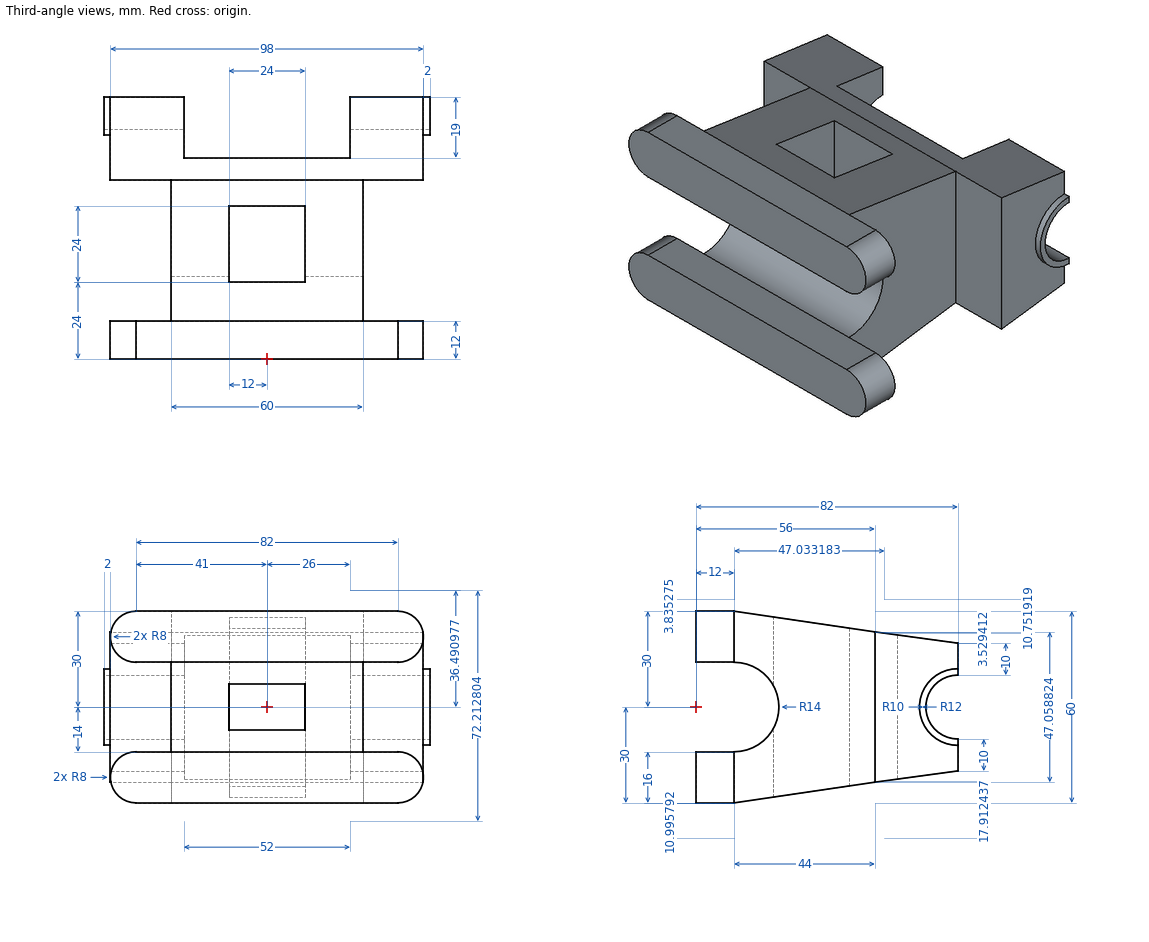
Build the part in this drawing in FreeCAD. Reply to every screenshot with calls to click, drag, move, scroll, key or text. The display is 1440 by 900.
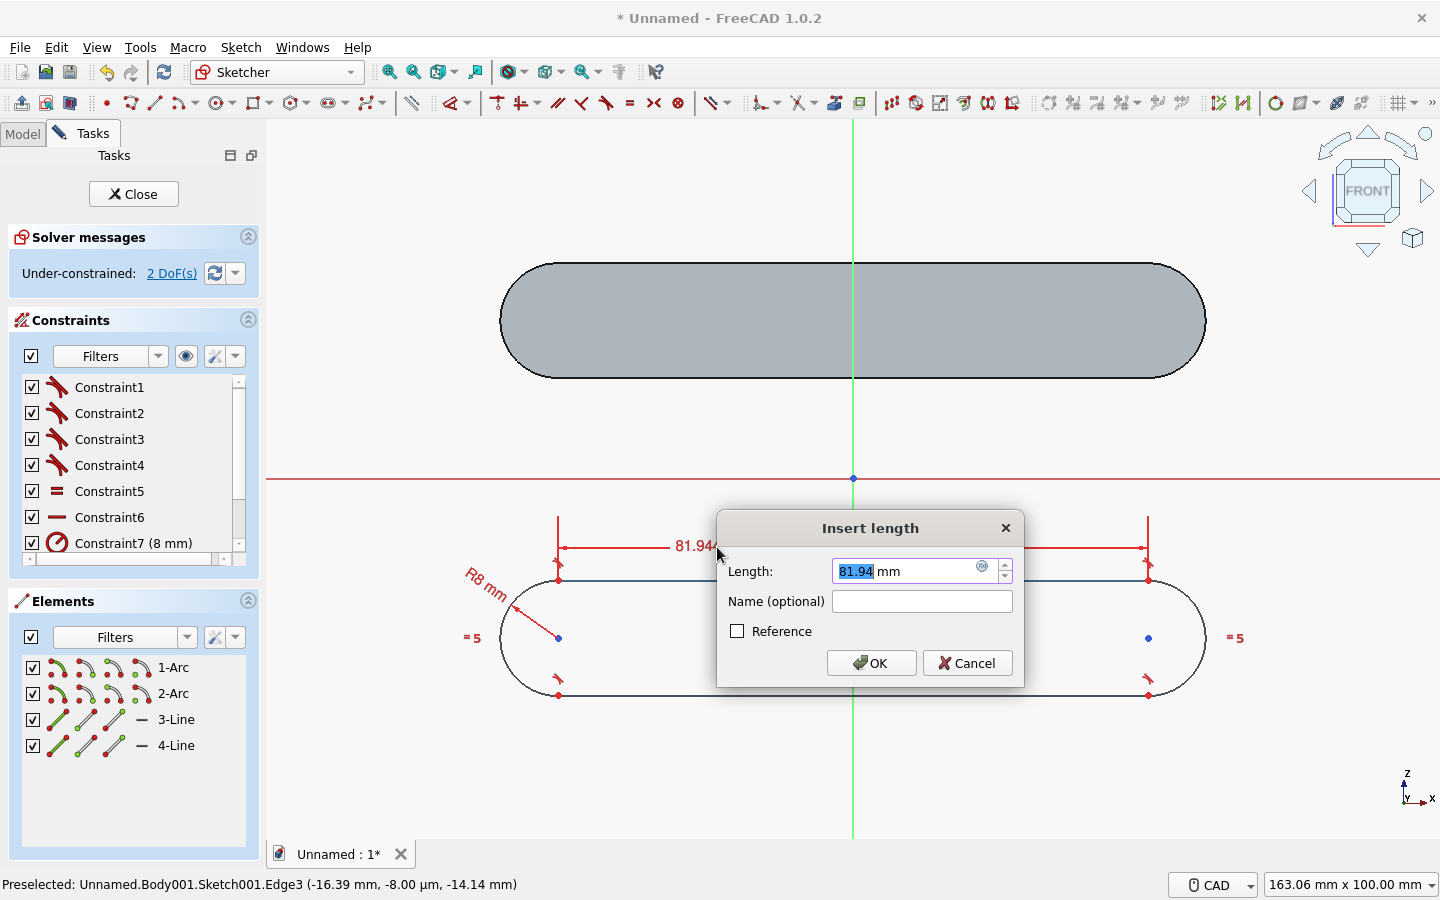
text(82)
key(Return)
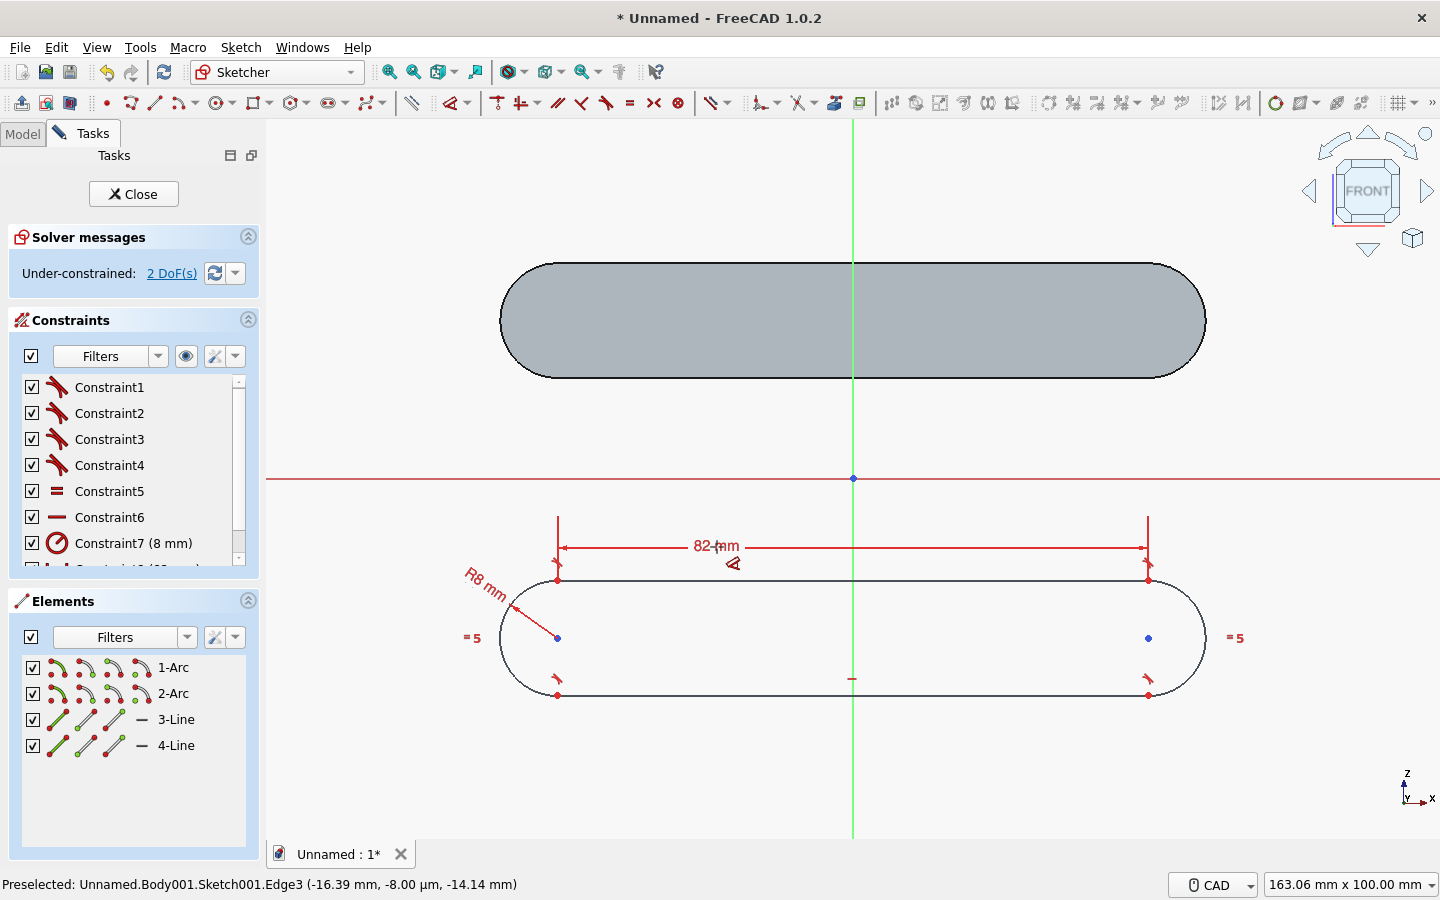
click(558, 581)
click(705, 445)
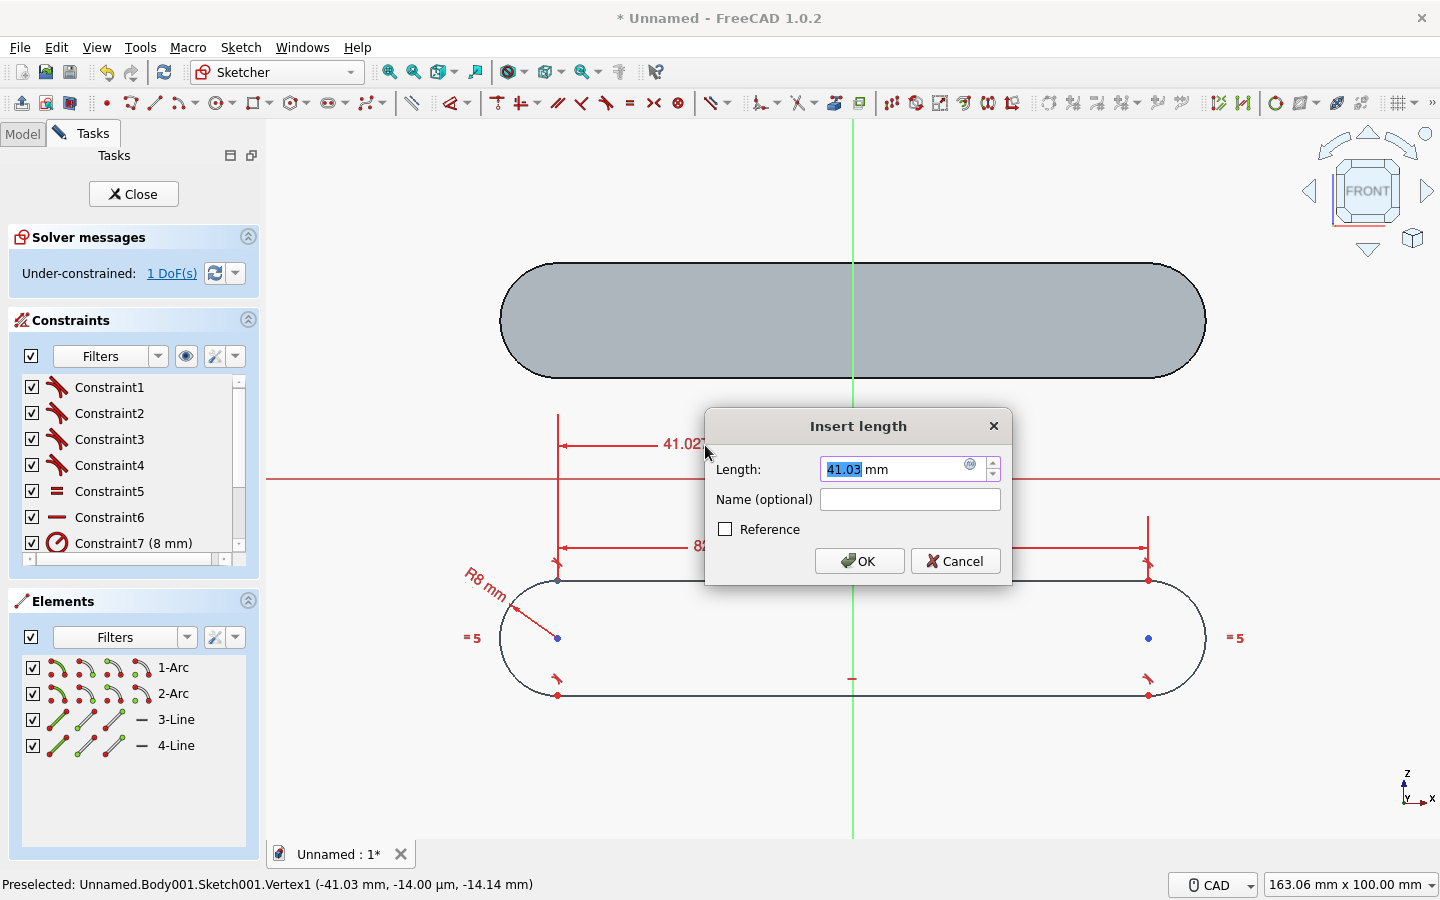
text(41)
key(Return)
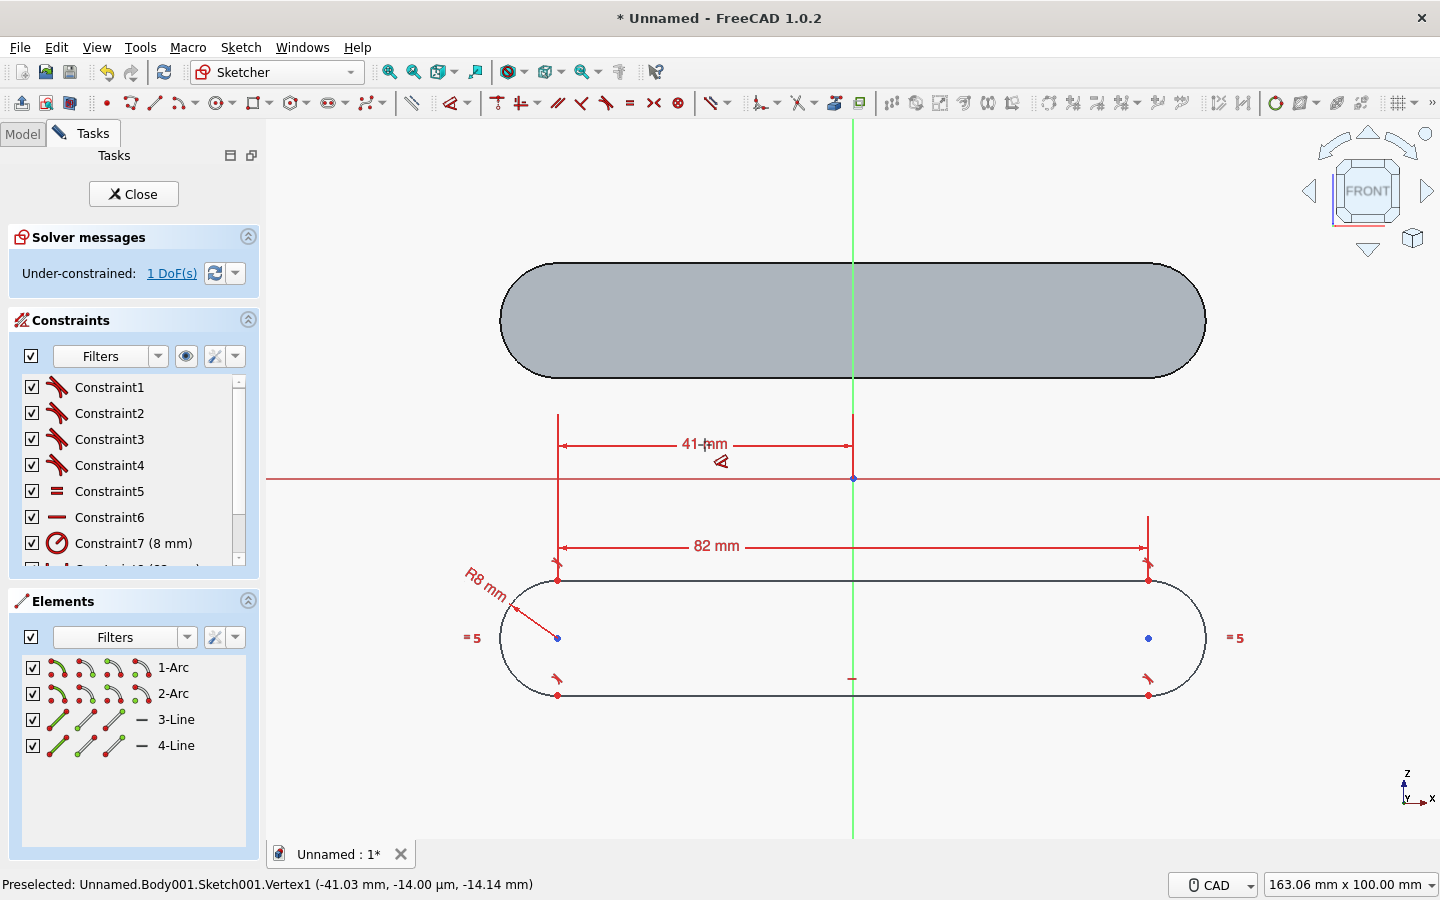
click(558, 581)
click(524, 530)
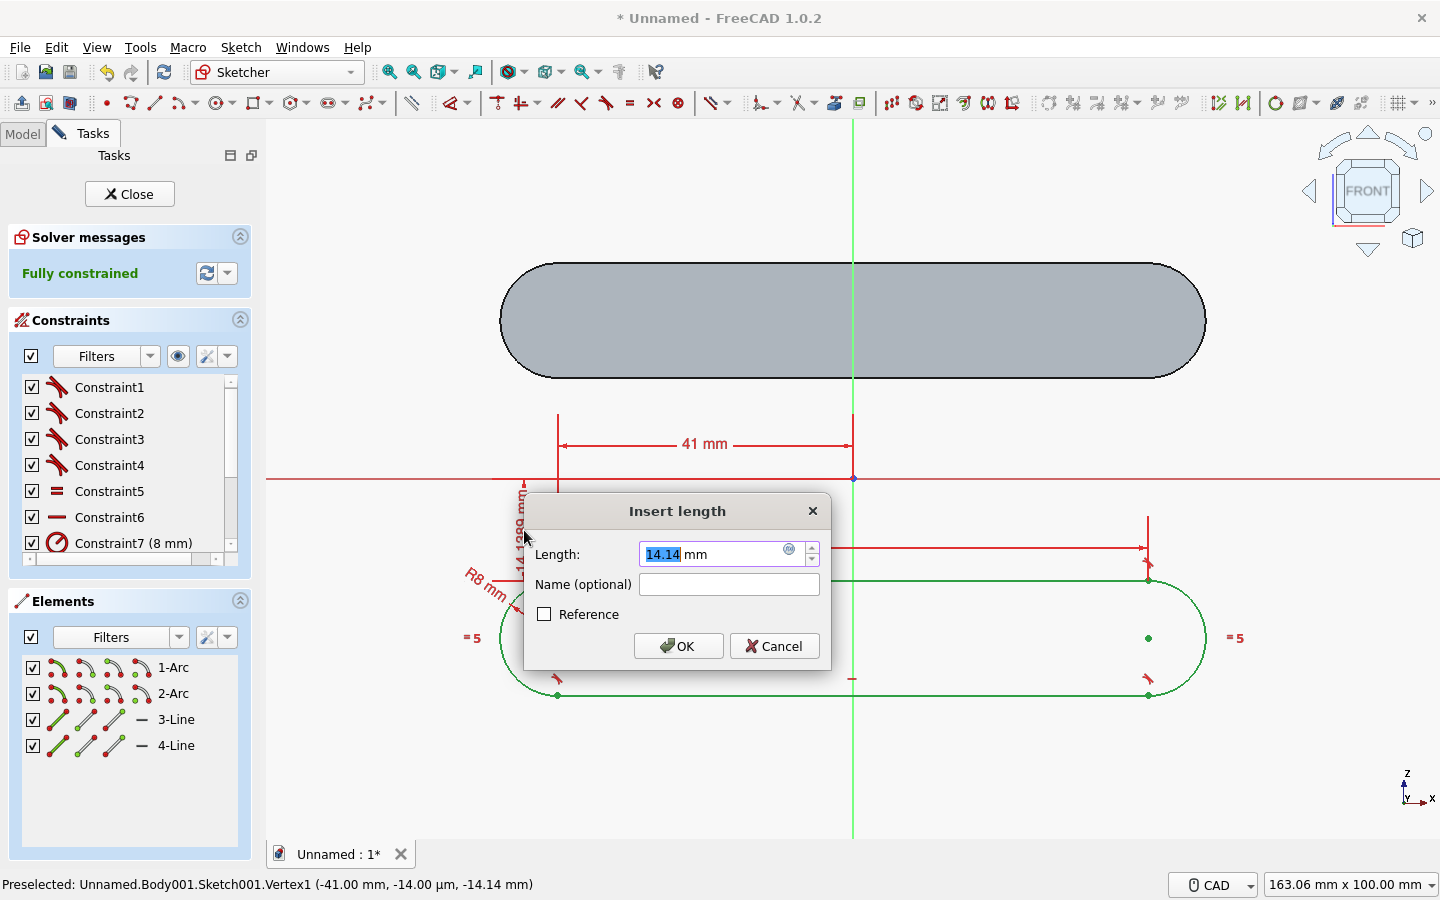
text(14)
key(Return)
key(Escape)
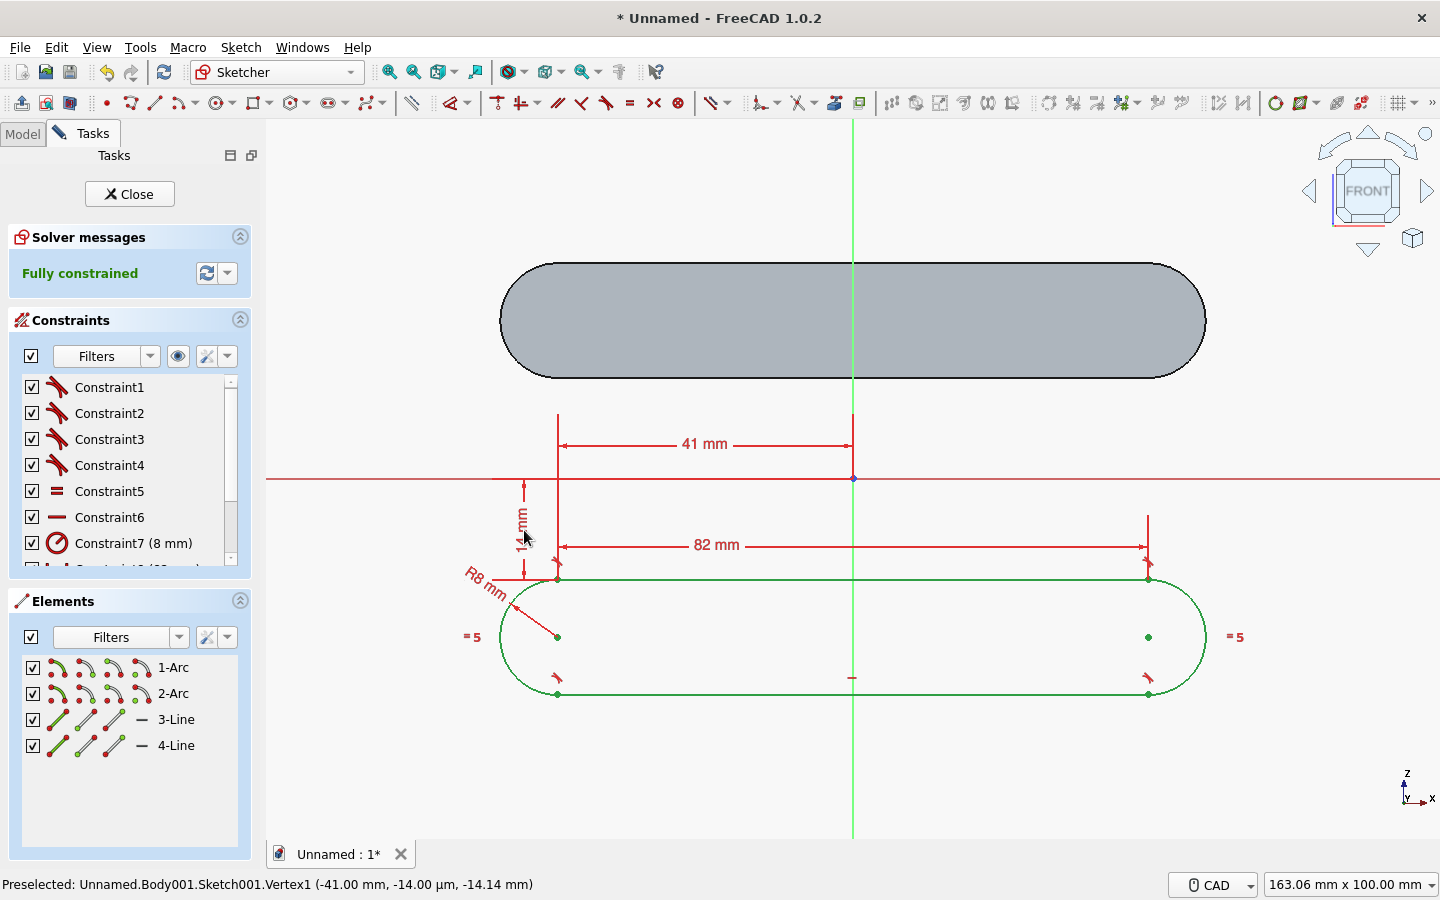
click(130, 194)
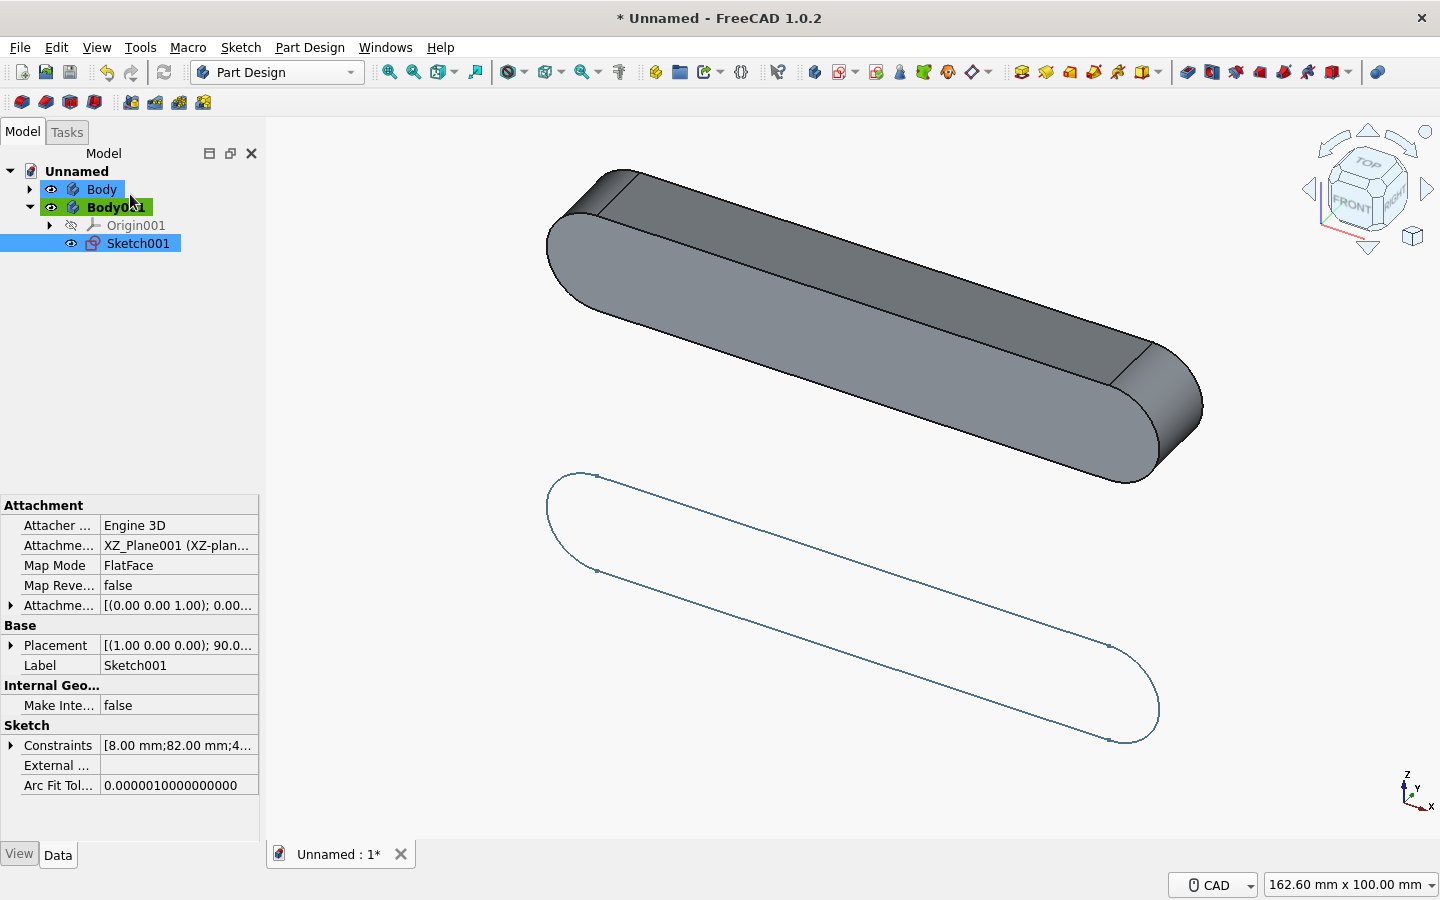
click(1022, 72)